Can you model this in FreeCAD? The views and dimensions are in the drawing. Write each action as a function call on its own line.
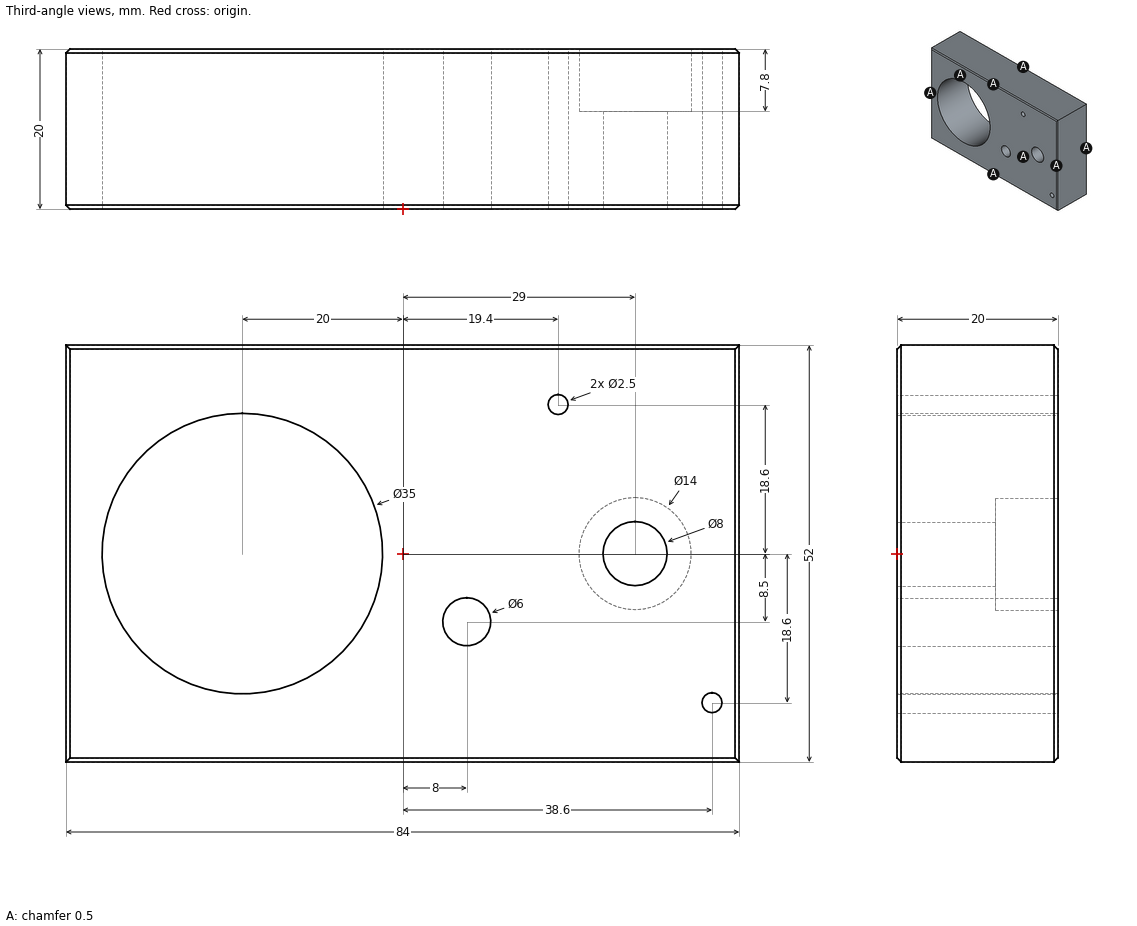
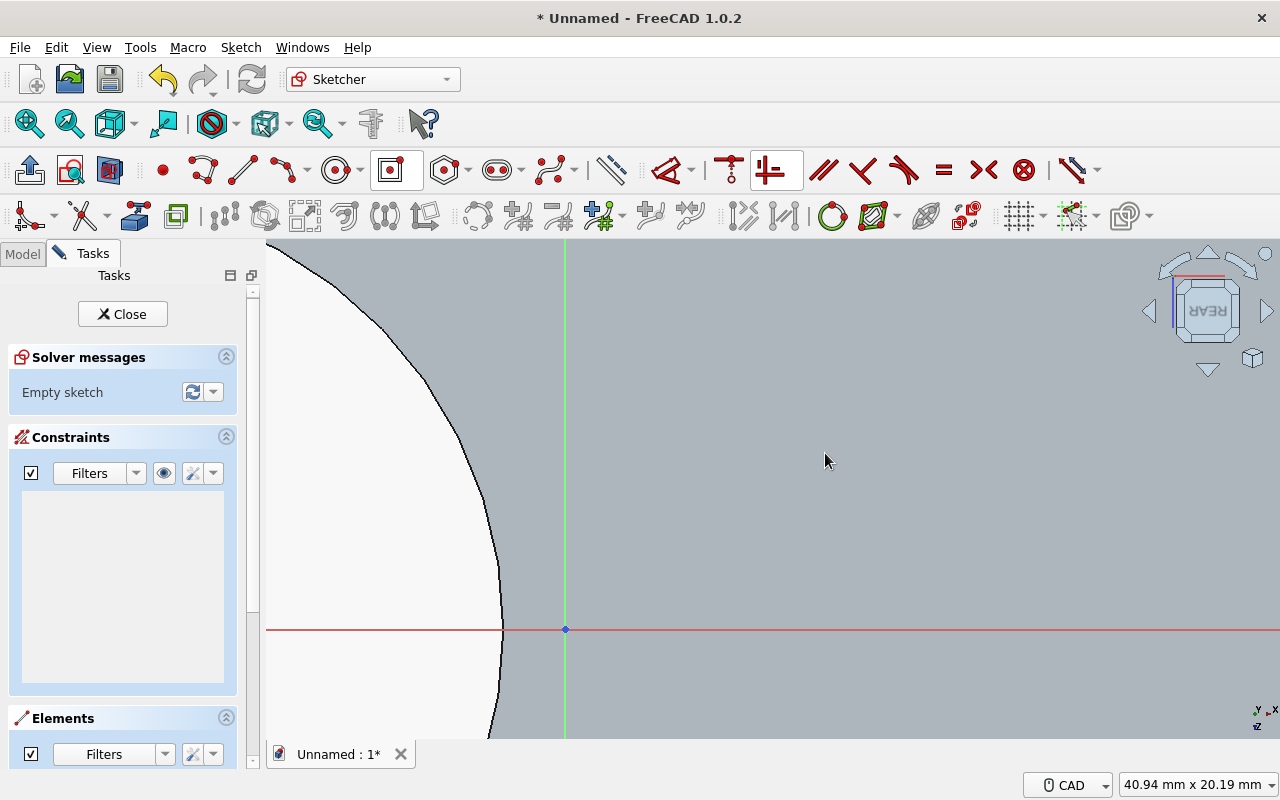
click(336, 170)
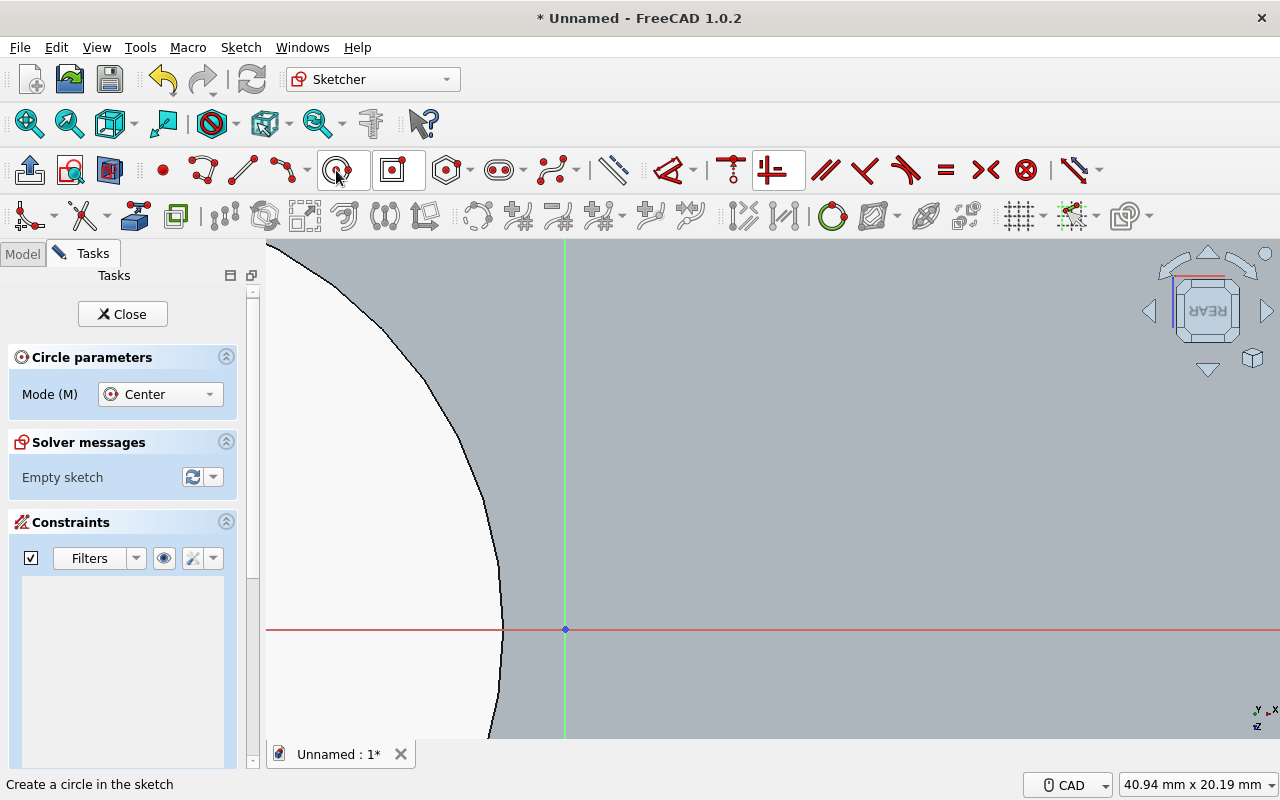
click(763, 419)
move(816, 367)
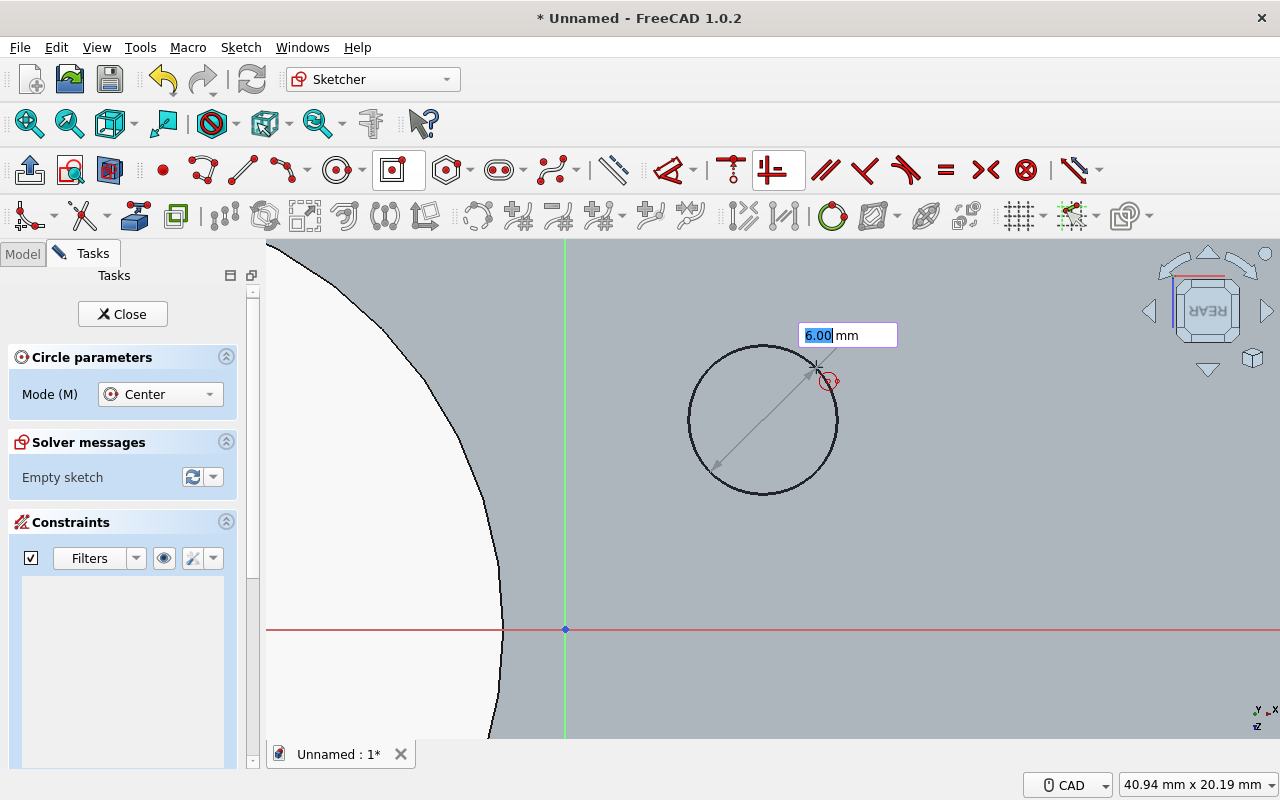
text(6)
key(Return)
key(Escape)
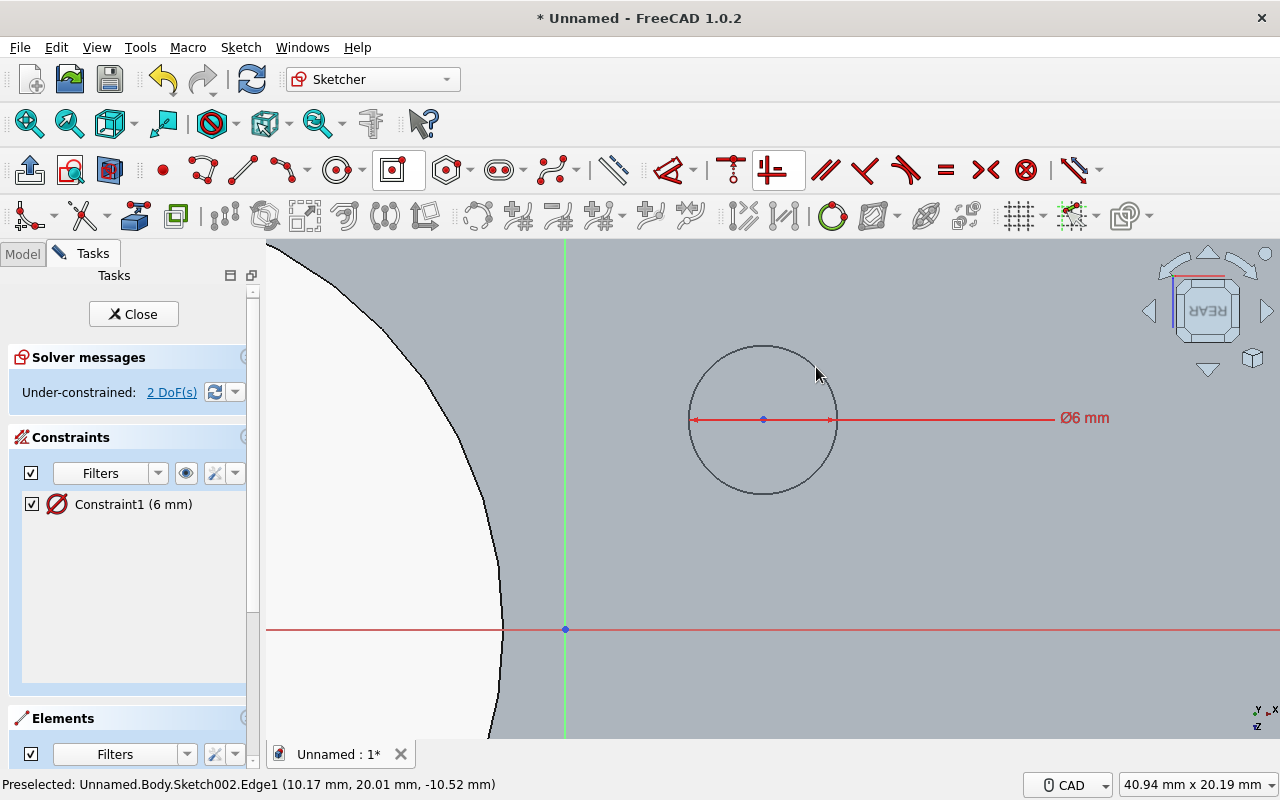
click(668, 170)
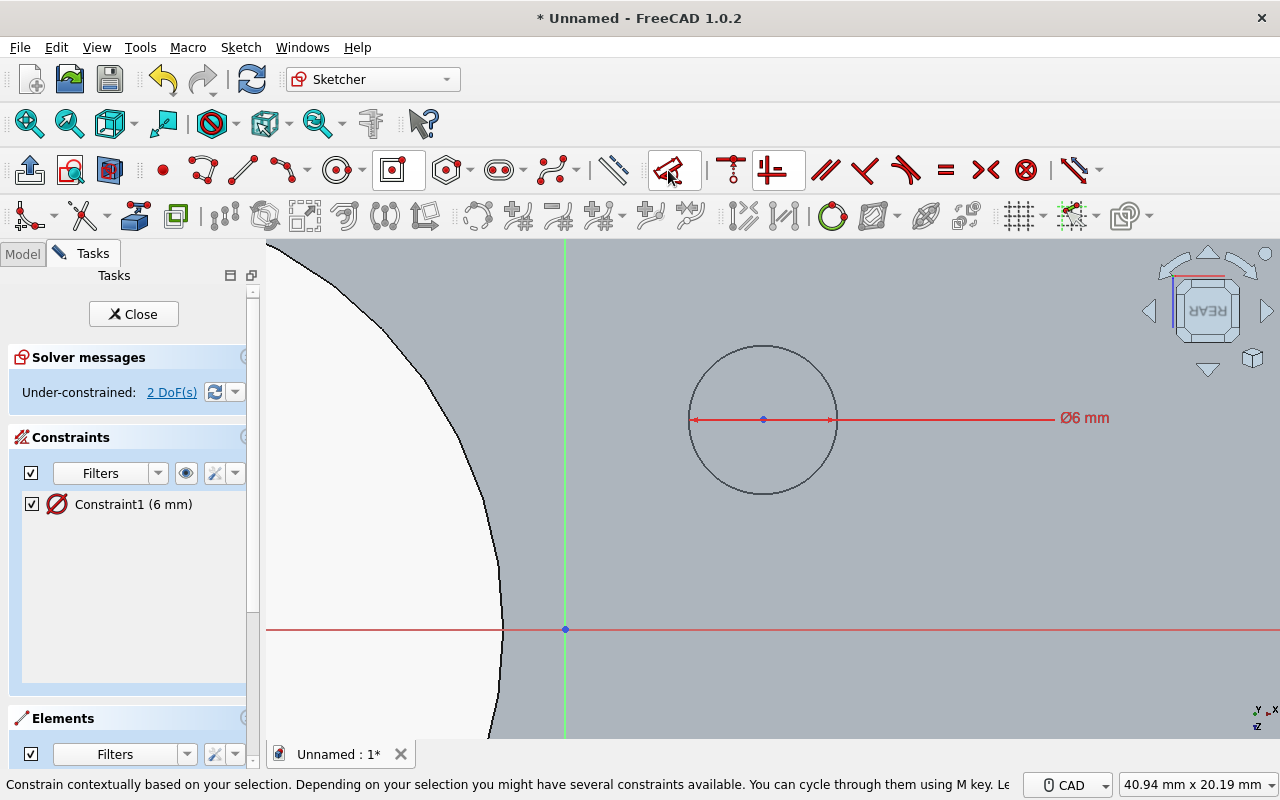
click(763, 420)
click(664, 664)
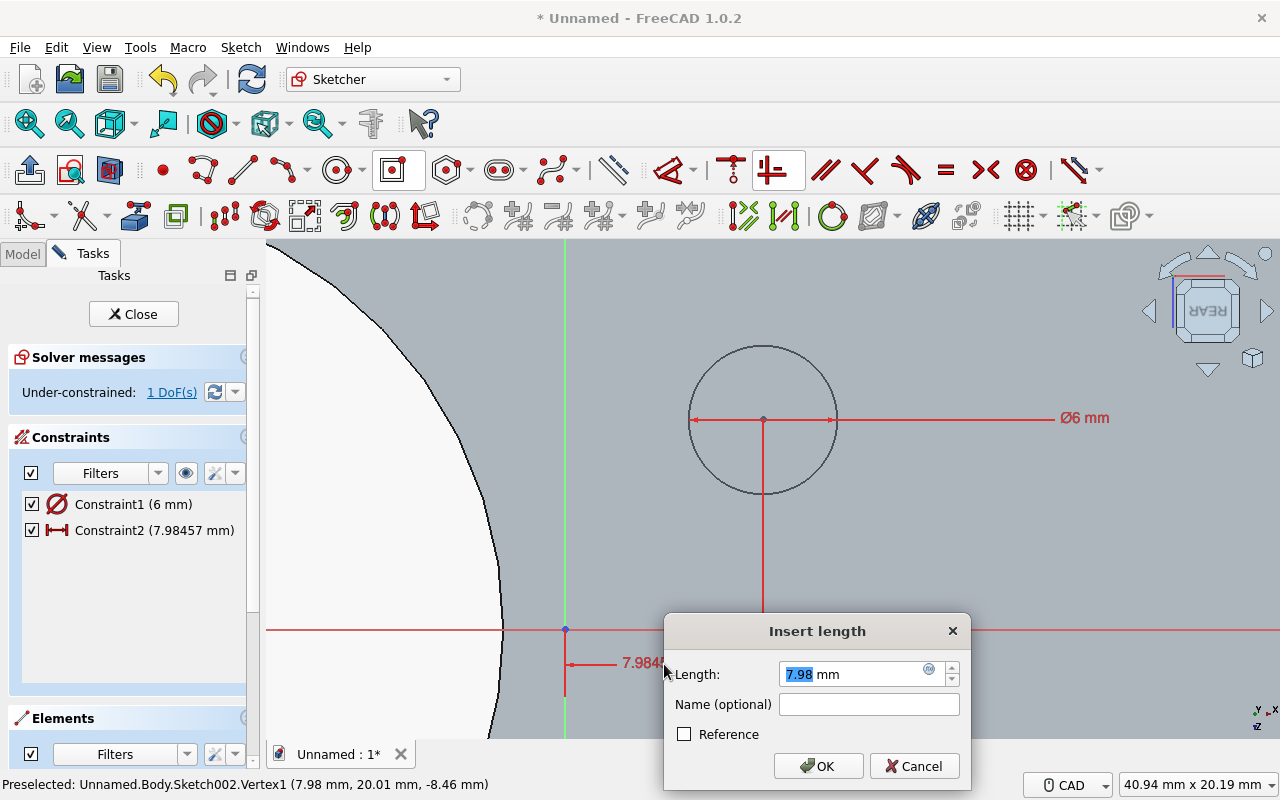
text(8)
key(Return)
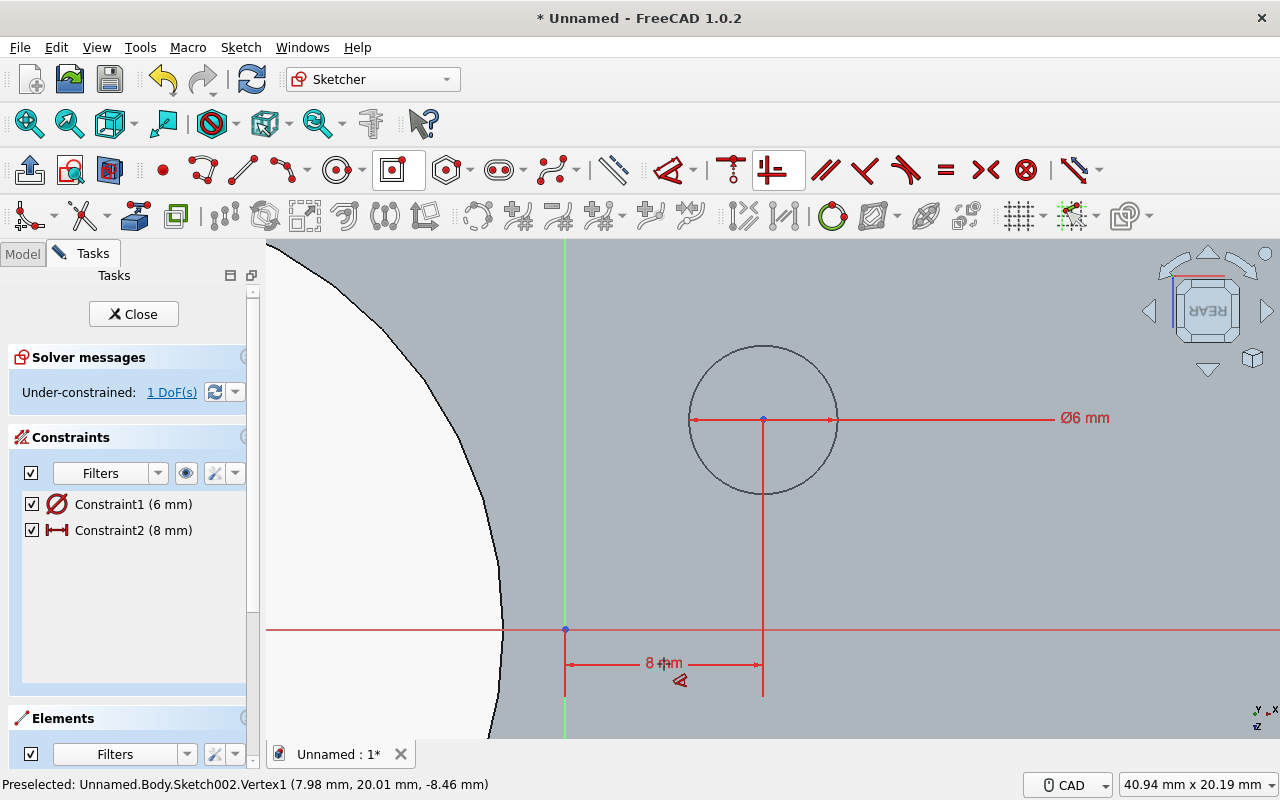
click(763, 420)
click(531, 525)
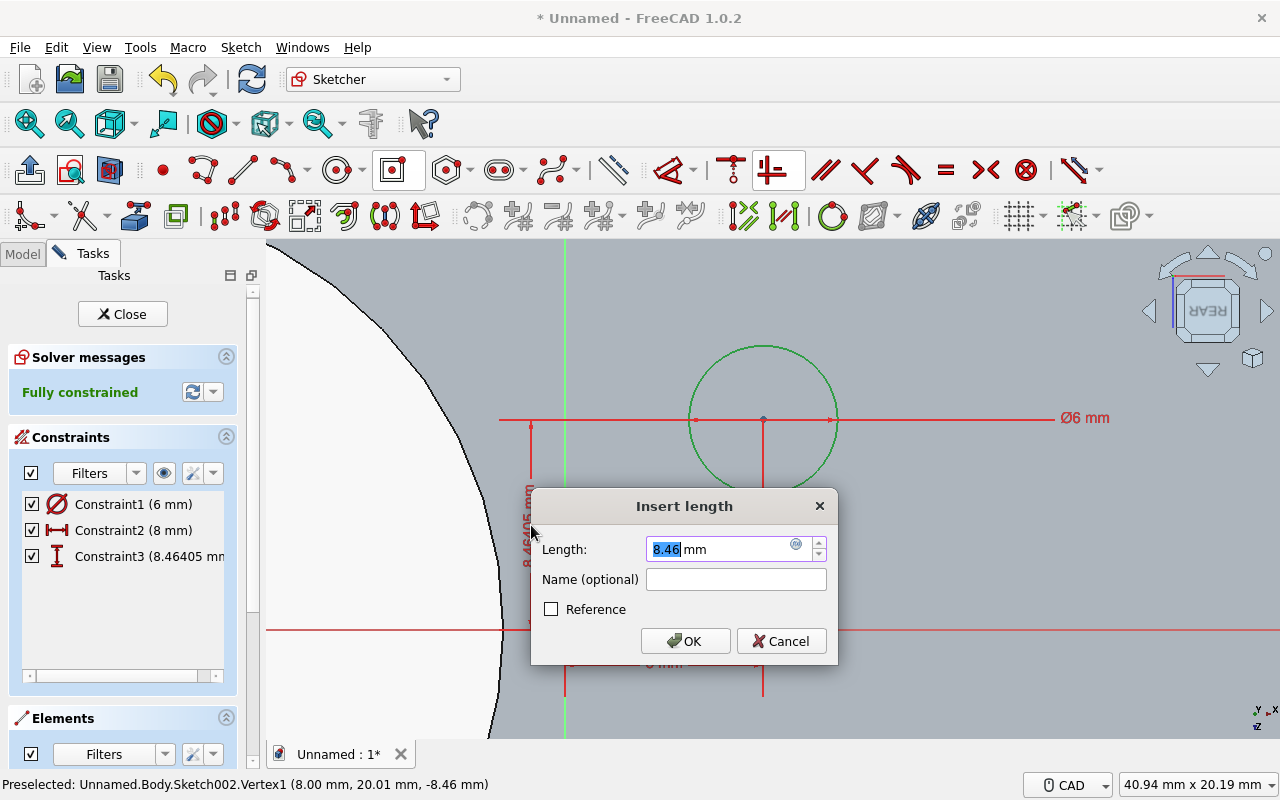
text(8.5)
key(Return)
key(Escape)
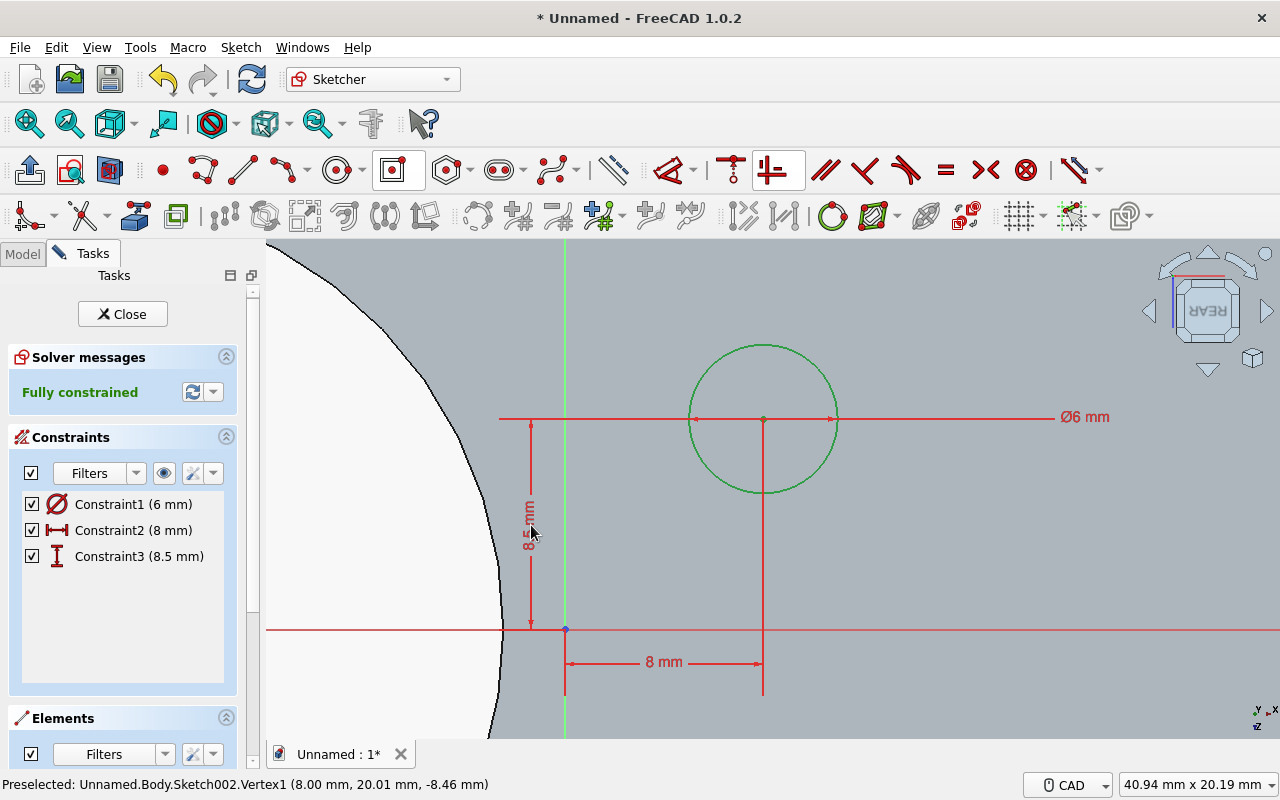
click(123, 314)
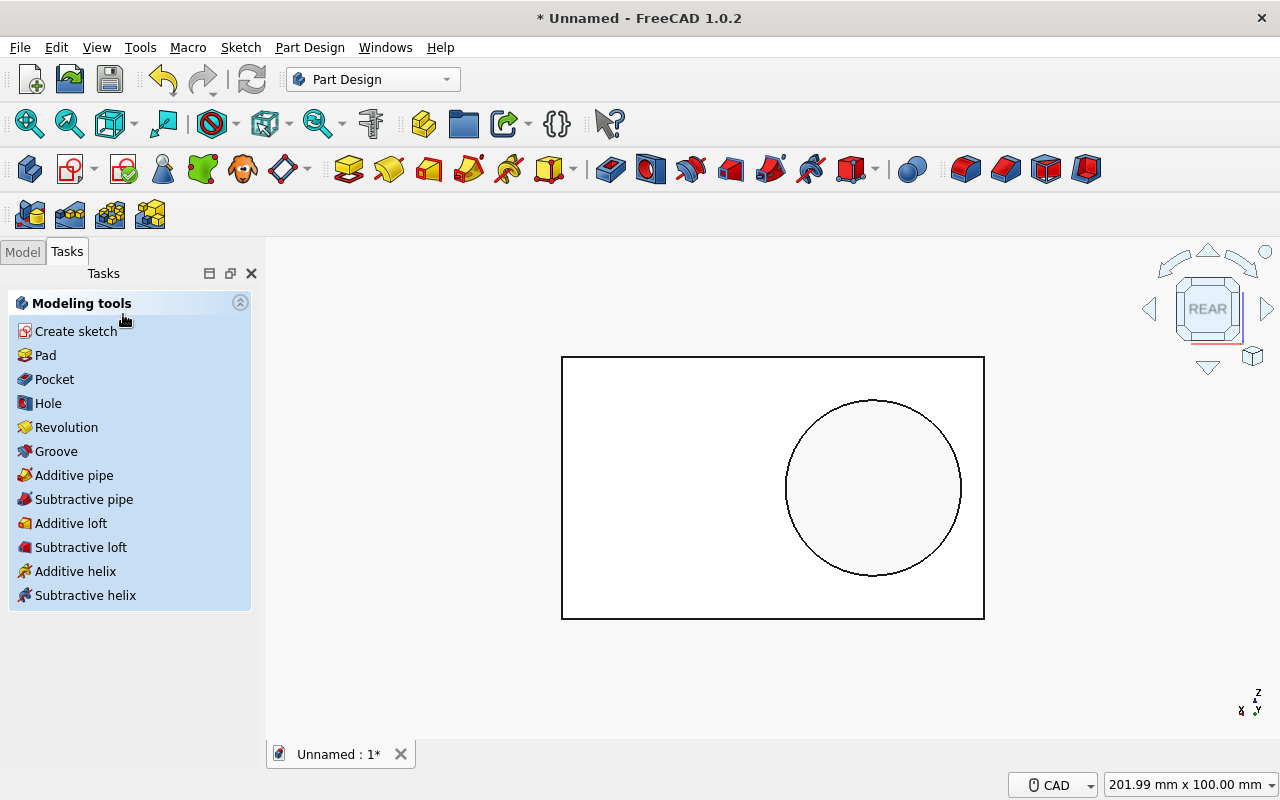
click(612, 170)